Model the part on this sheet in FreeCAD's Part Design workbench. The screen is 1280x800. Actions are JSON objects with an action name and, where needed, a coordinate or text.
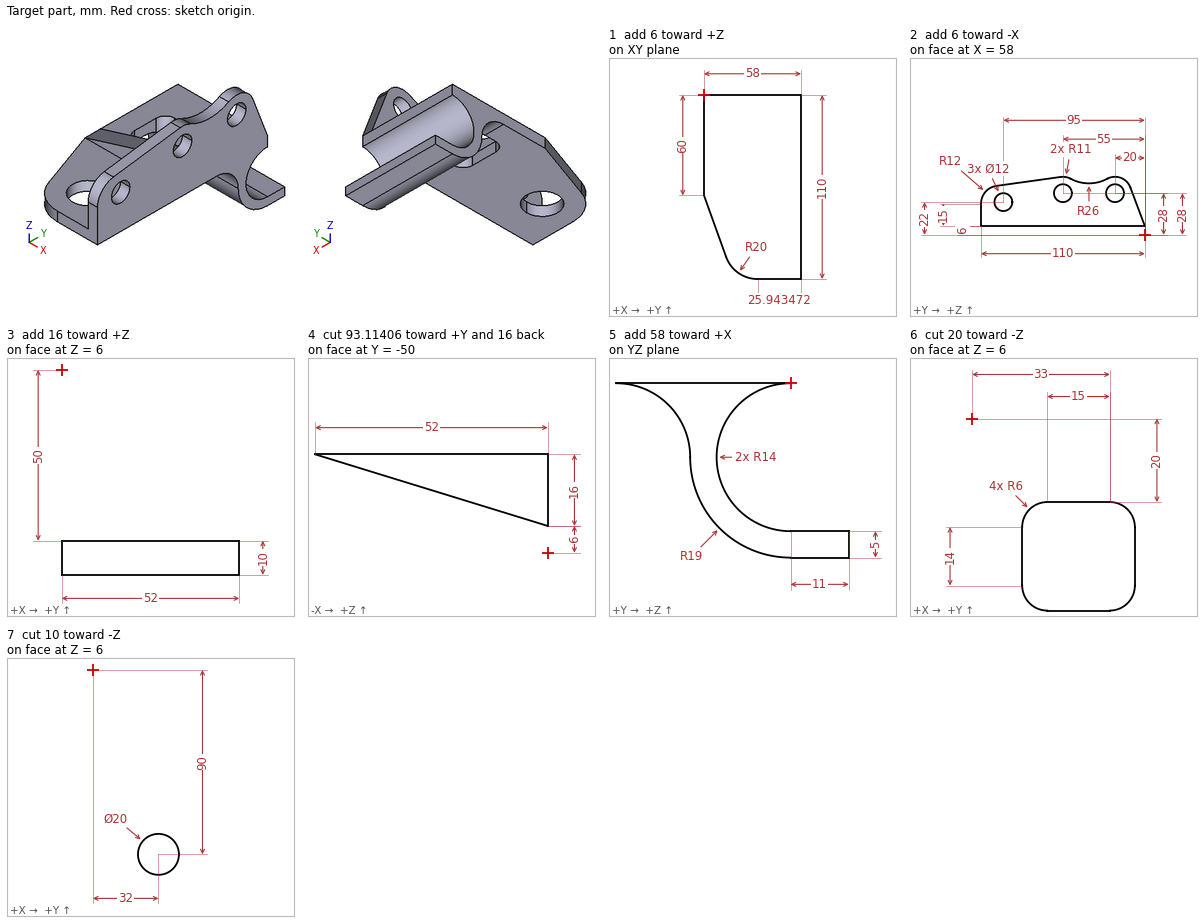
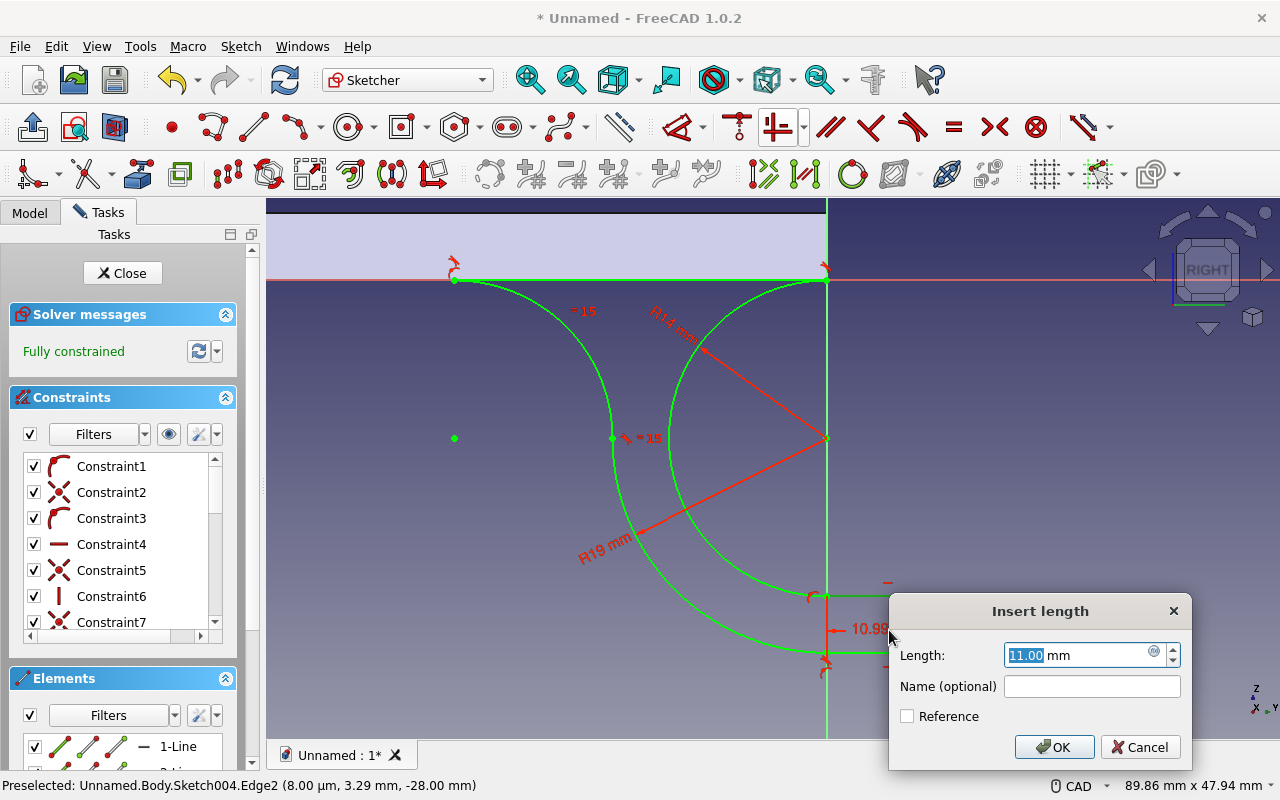
{"action": "type", "text": "11"}
{"action": "key", "text": "Return"}
{"action": "key", "text": "Escape"}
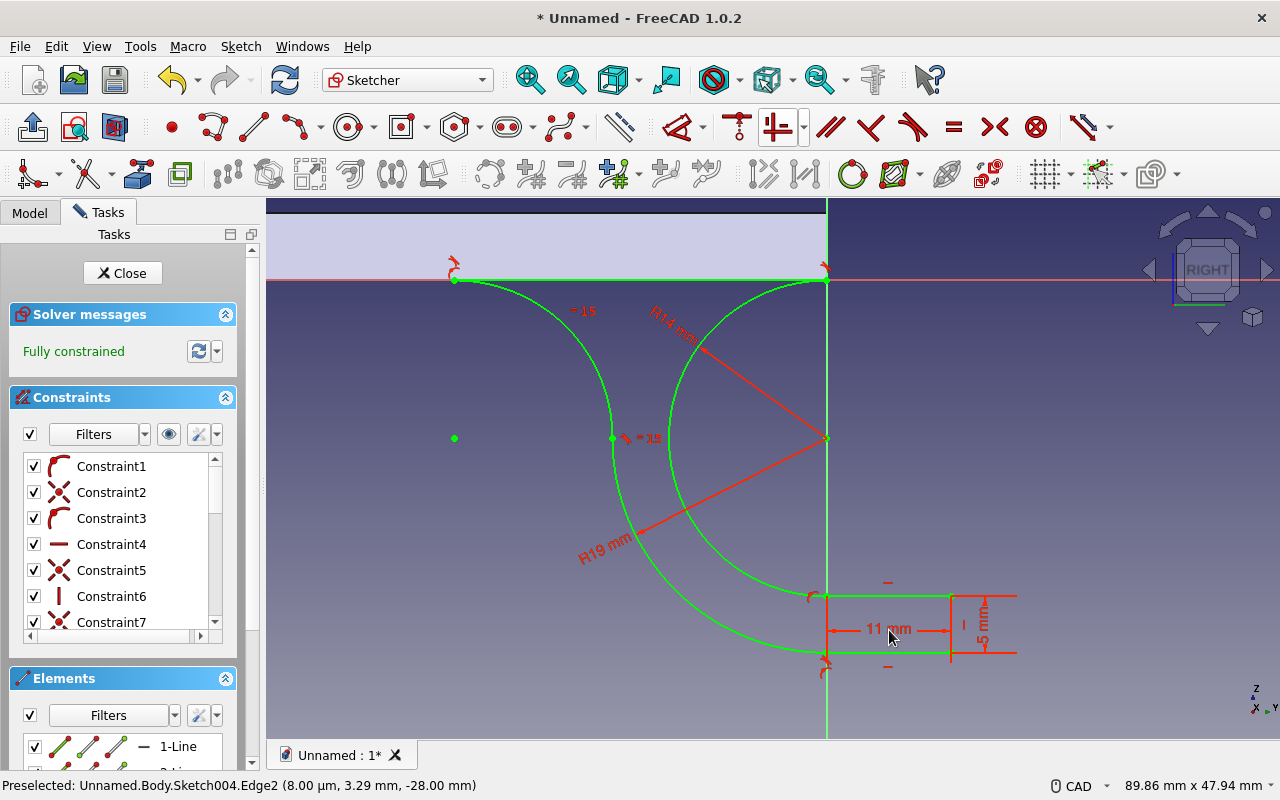
{"action": "left_click", "coordinate": [123, 273]}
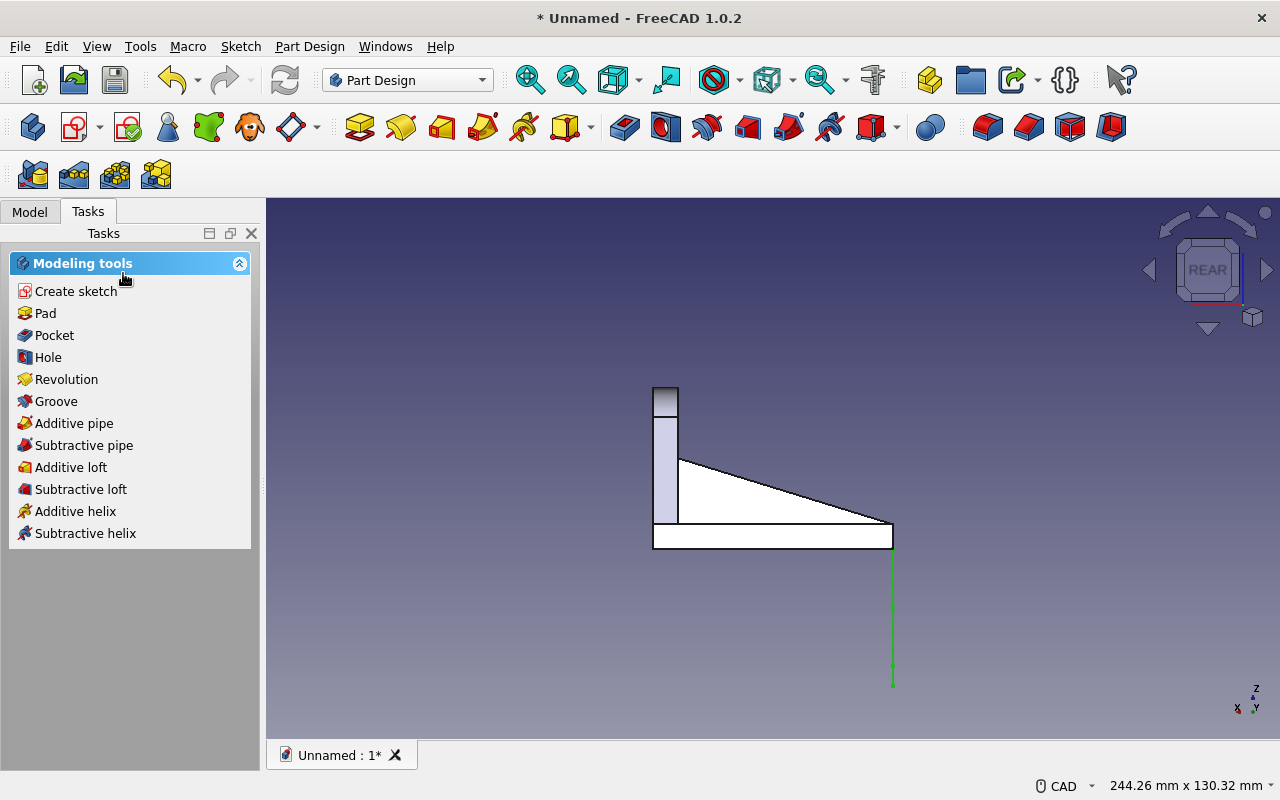
{"action": "left_click", "coordinate": [360, 128]}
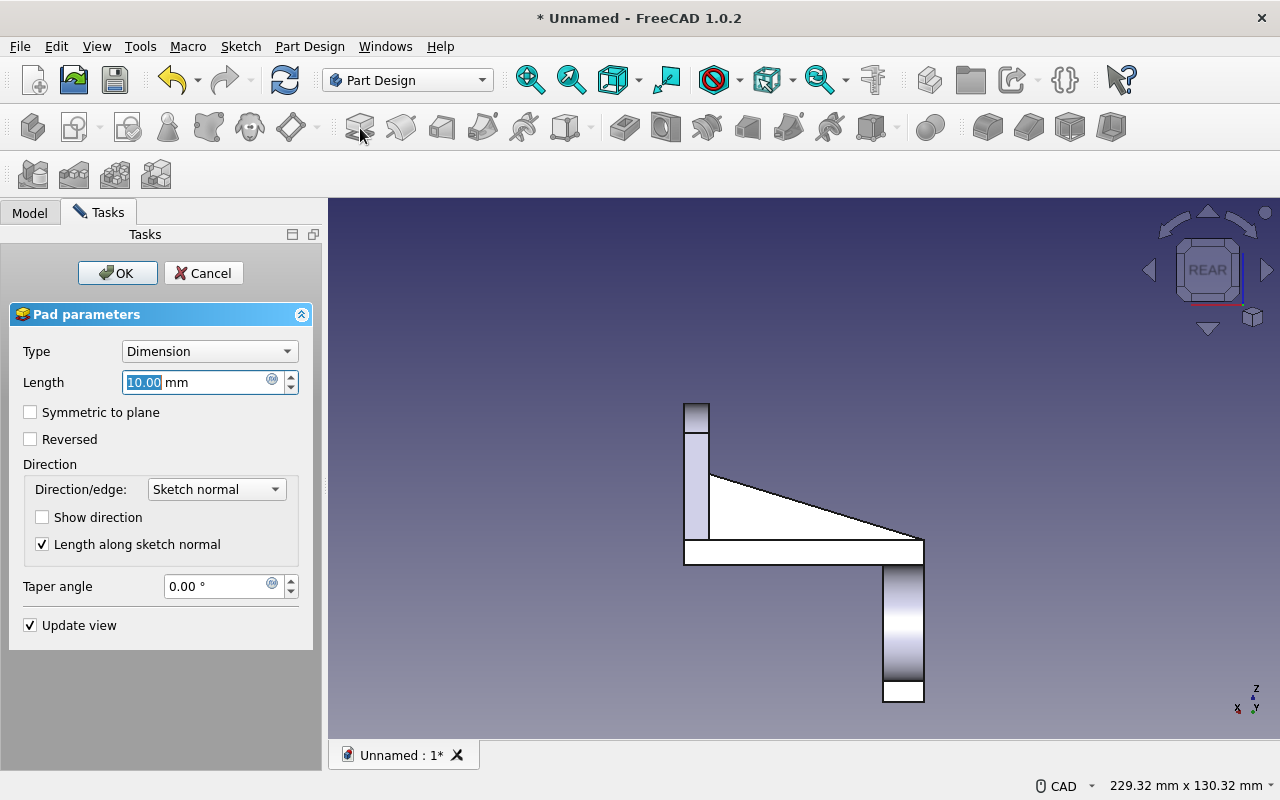
{"action": "type", "text": "58"}
{"action": "key", "text": "Tab"}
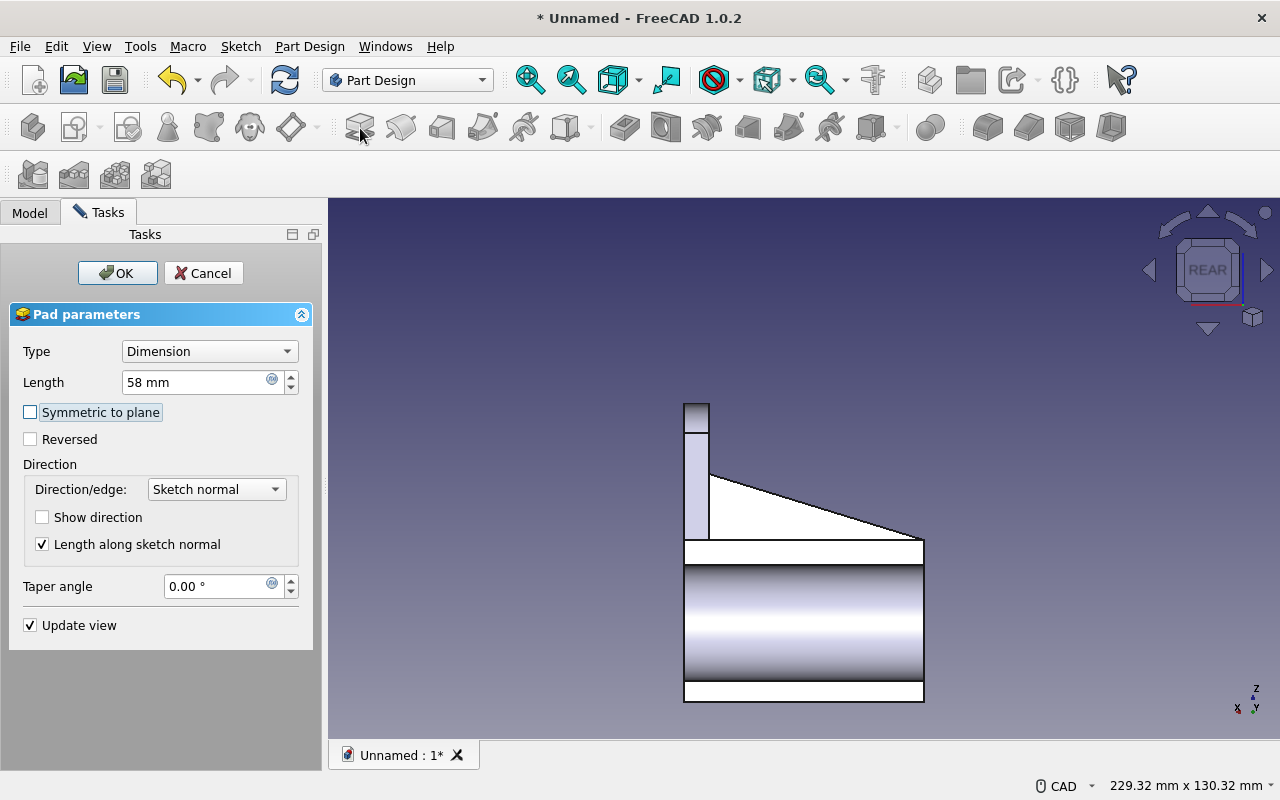
{"action": "left_click", "coordinate": [118, 273]}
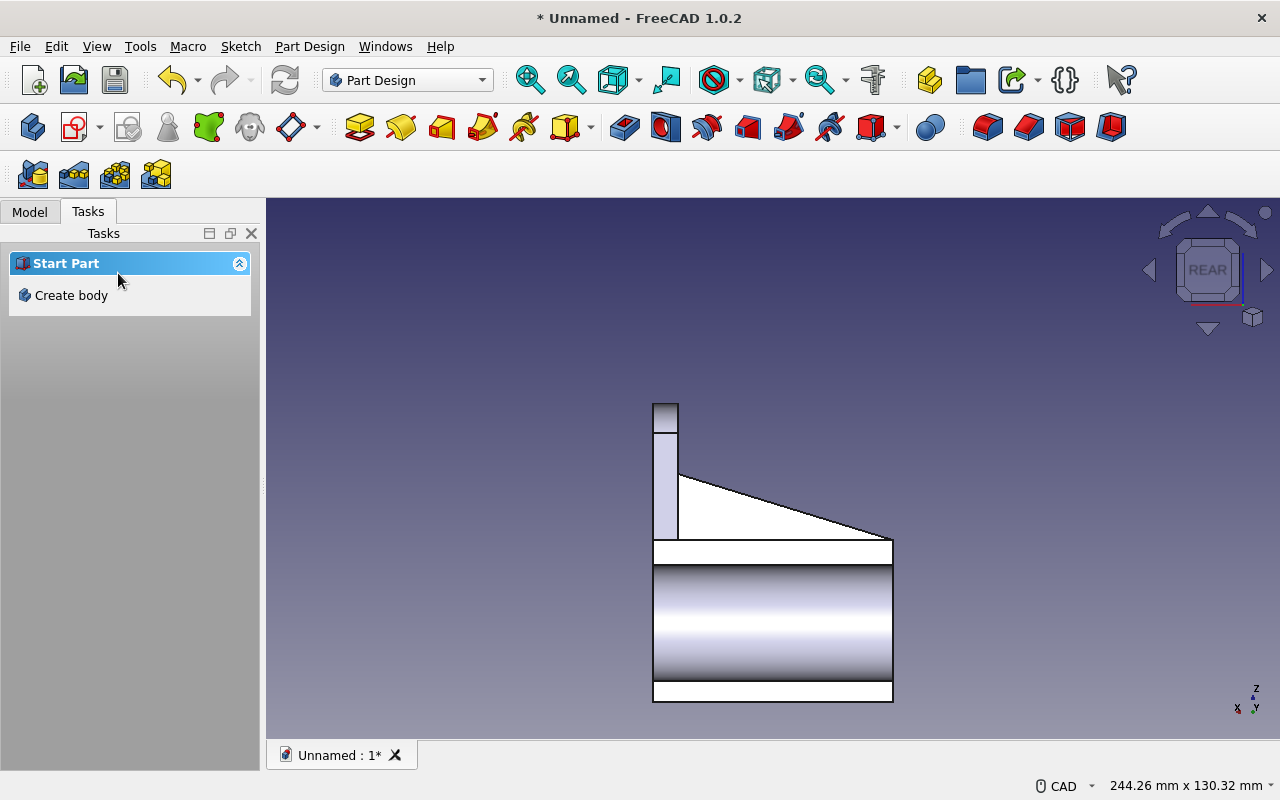
{"action": "key", "text": "0"}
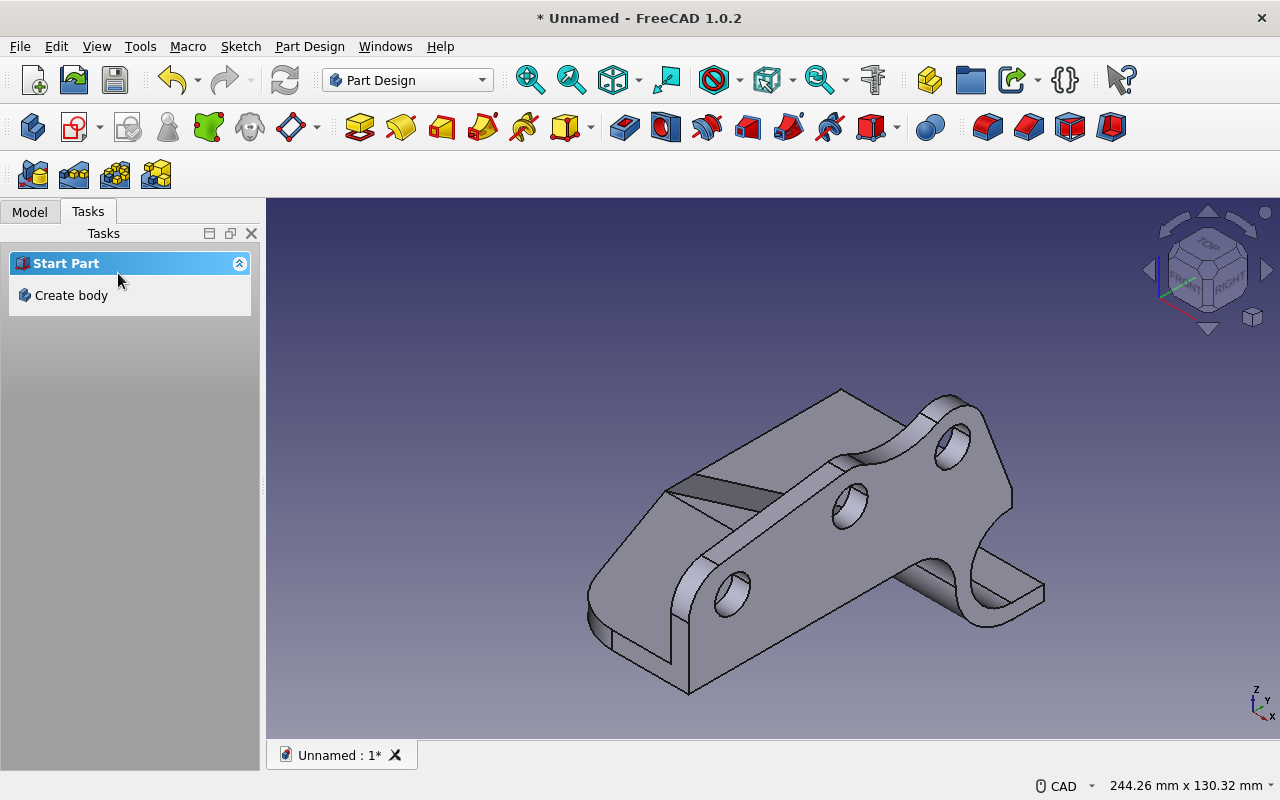
{"action": "left_click", "coordinate": [531, 80]}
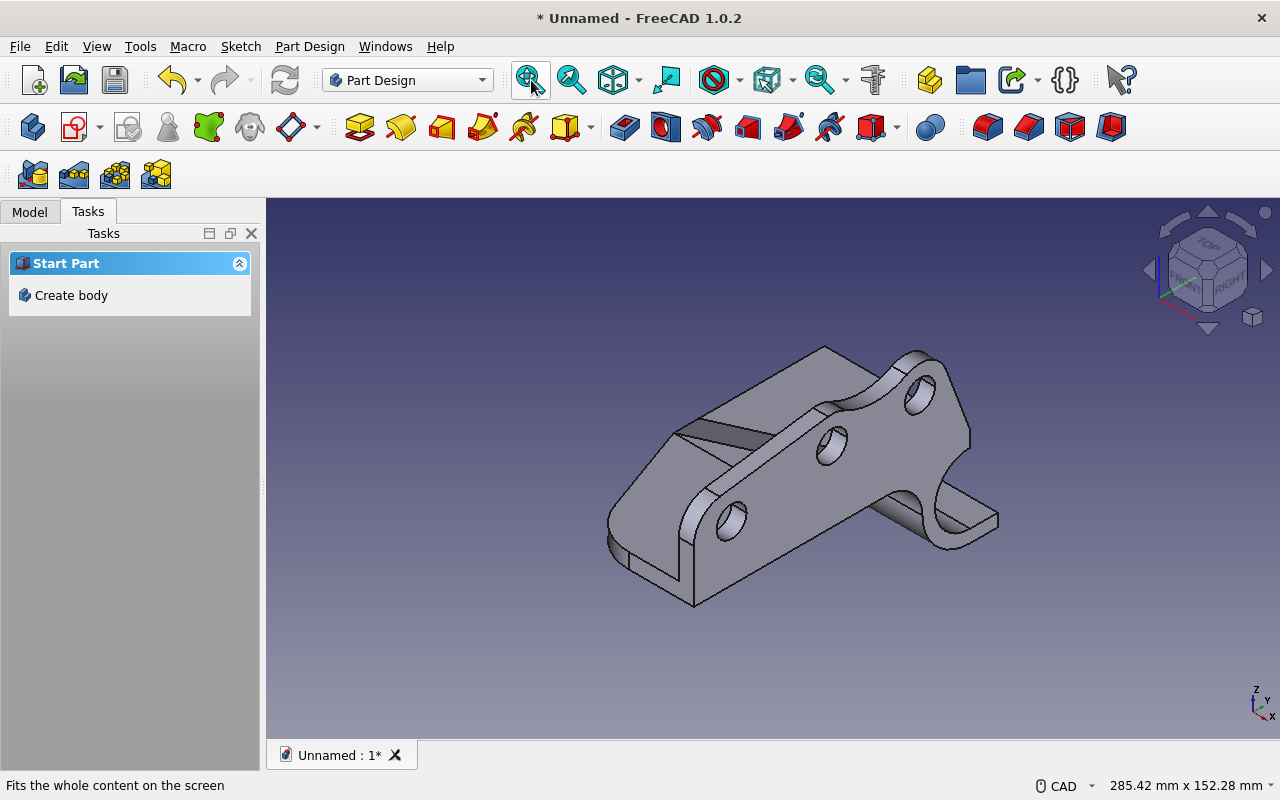
{"action": "key", "text": "2"}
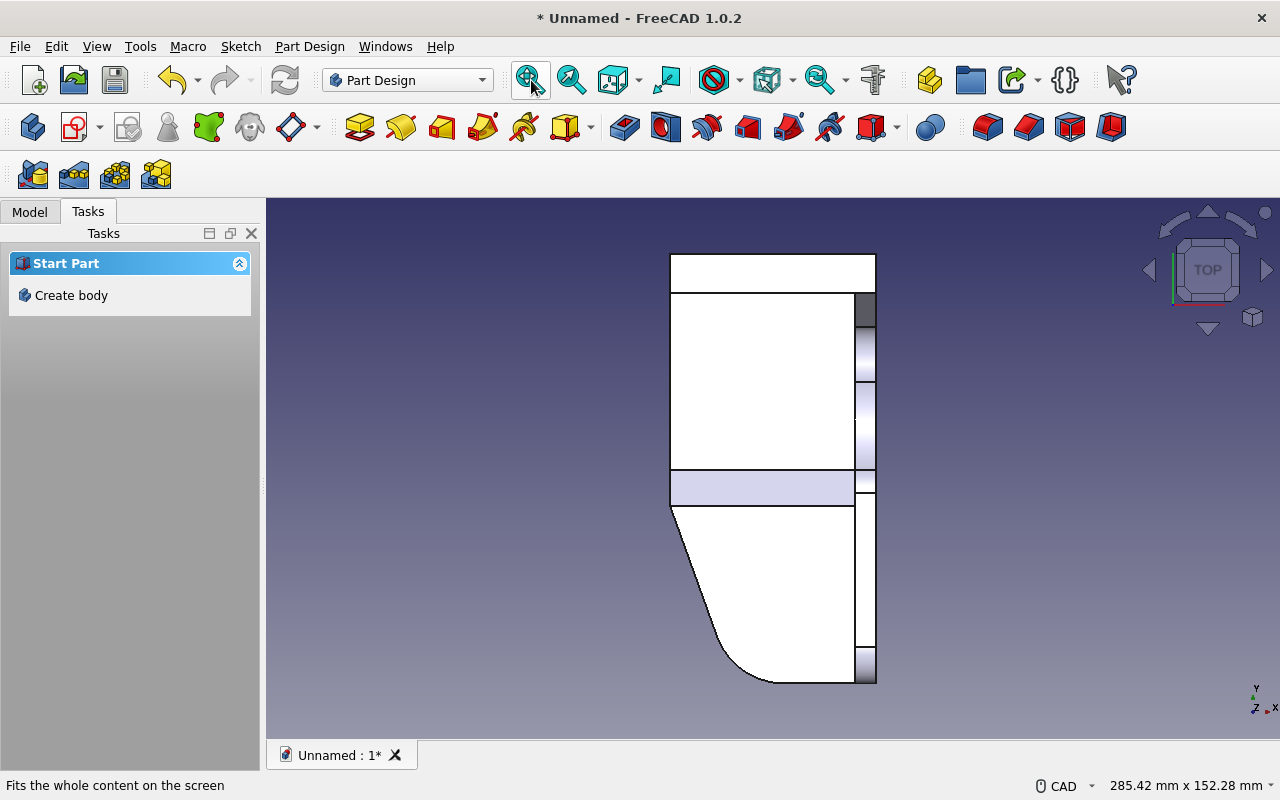
{"action": "left_click", "coordinate": [762, 380]}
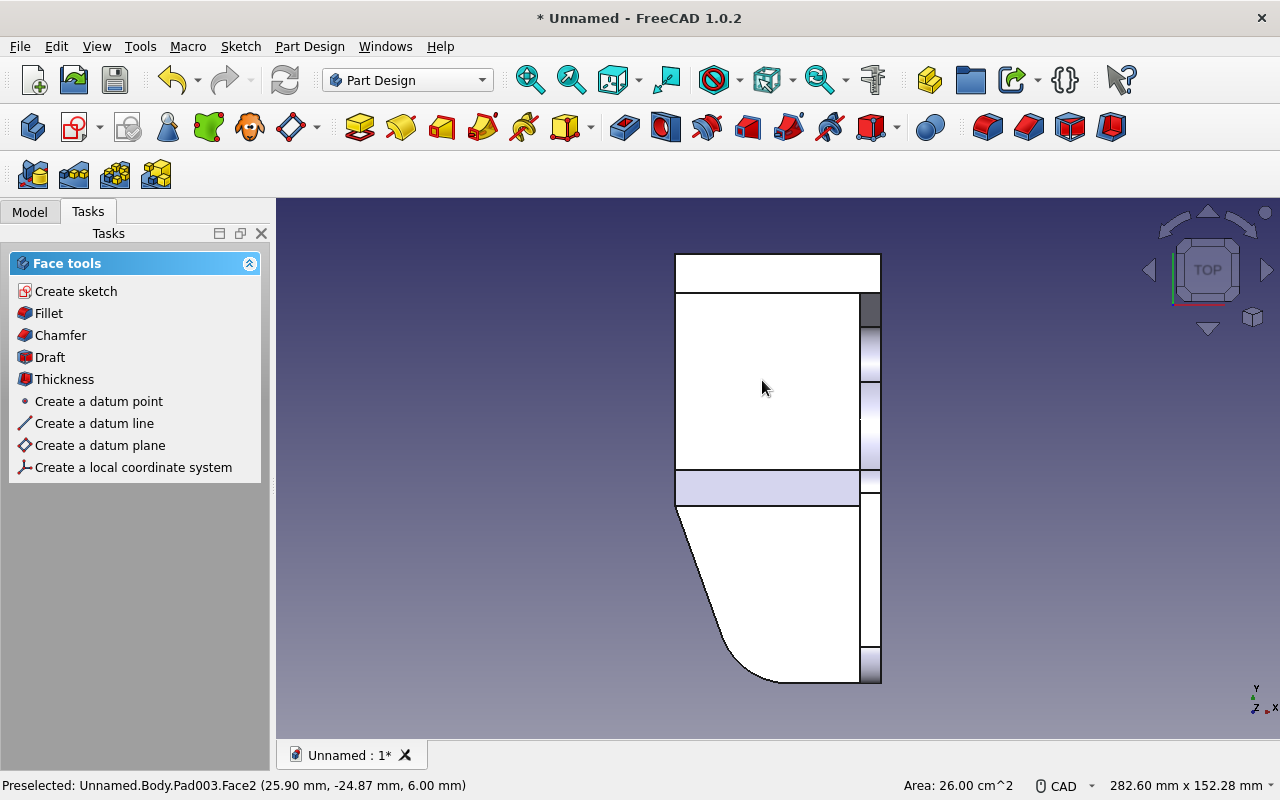
{"action": "left_click", "coordinate": [74, 128]}